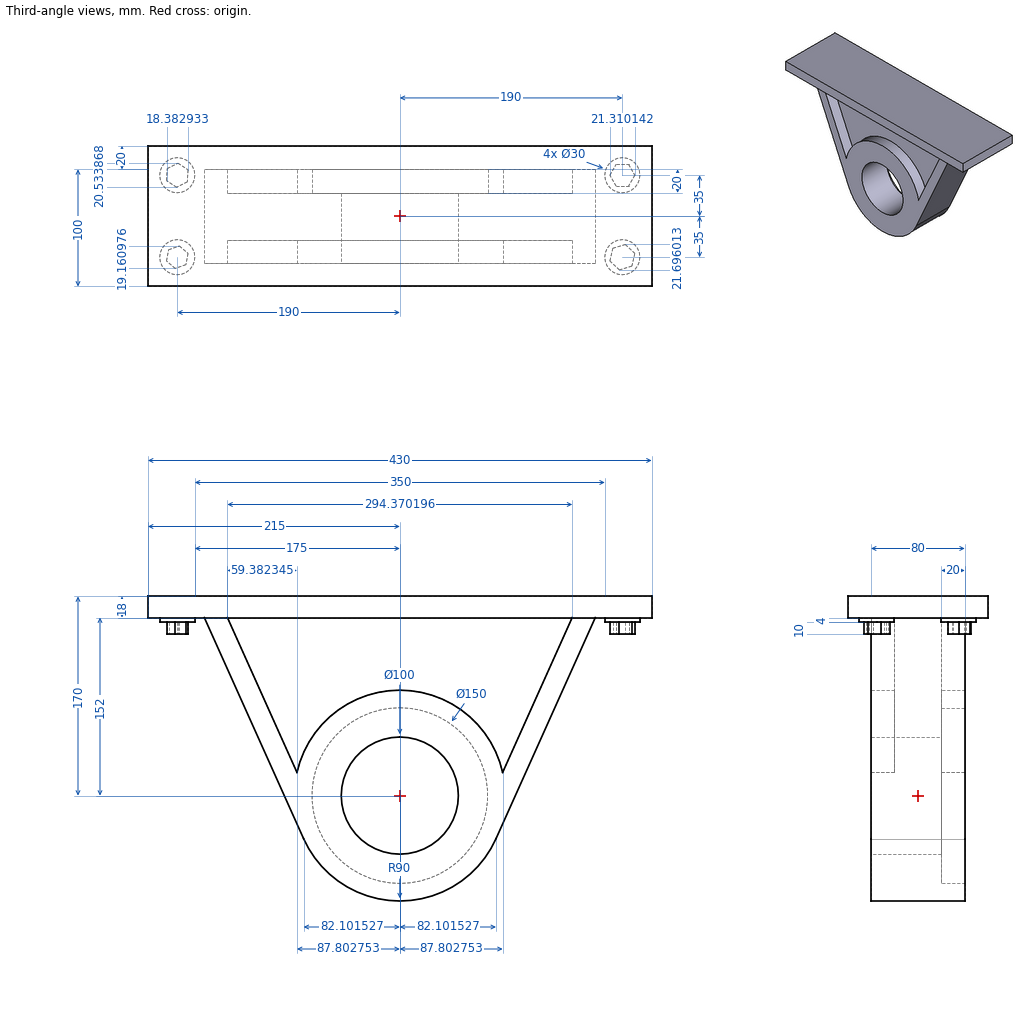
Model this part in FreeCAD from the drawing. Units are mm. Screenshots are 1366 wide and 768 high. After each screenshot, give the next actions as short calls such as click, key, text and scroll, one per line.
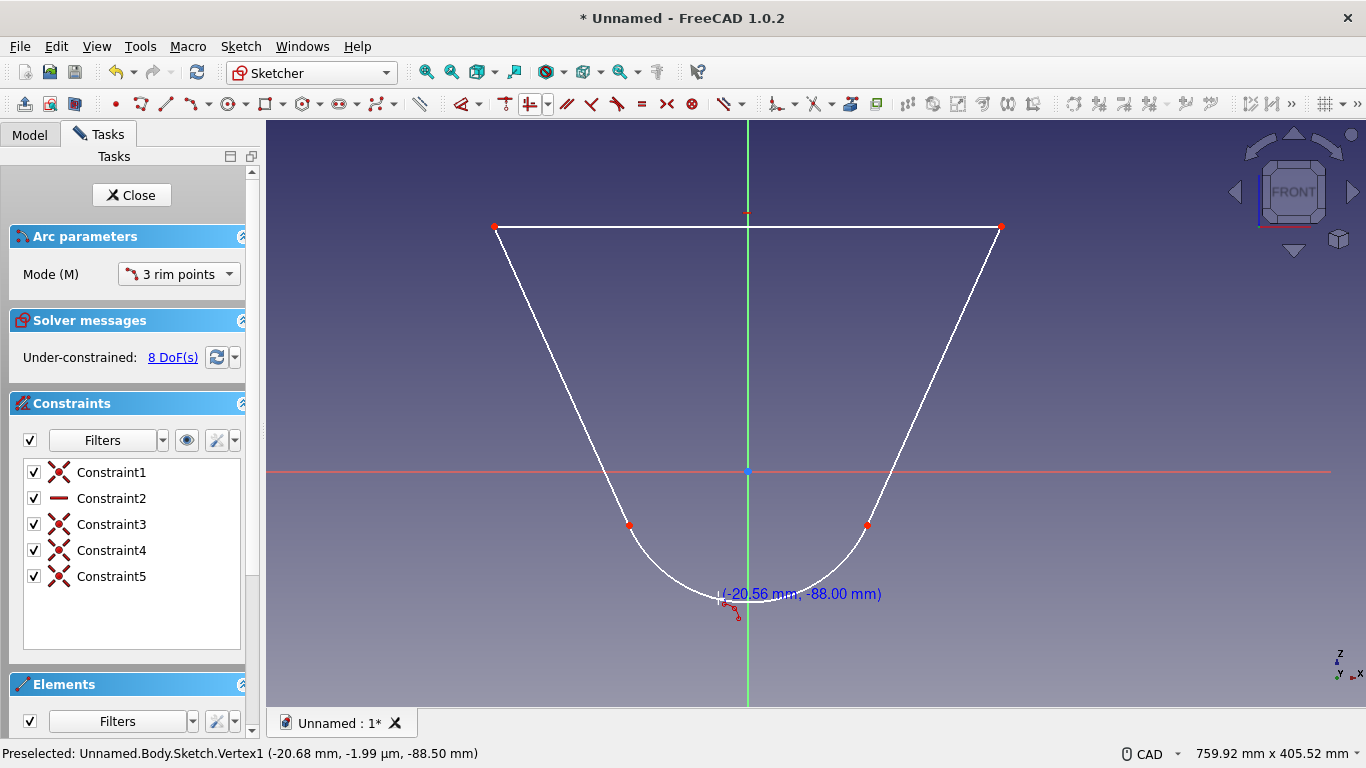
click(228, 104)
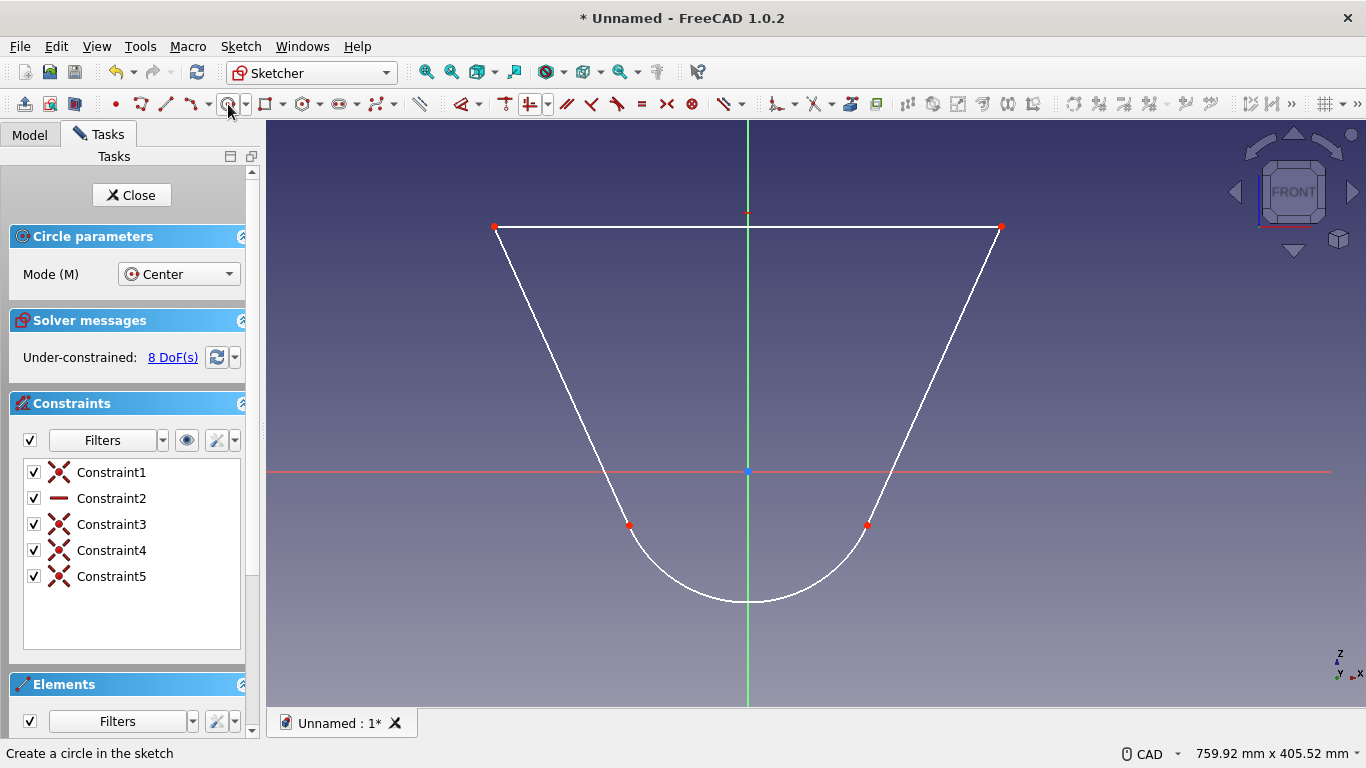
click(748, 472)
click(799, 420)
key(Escape)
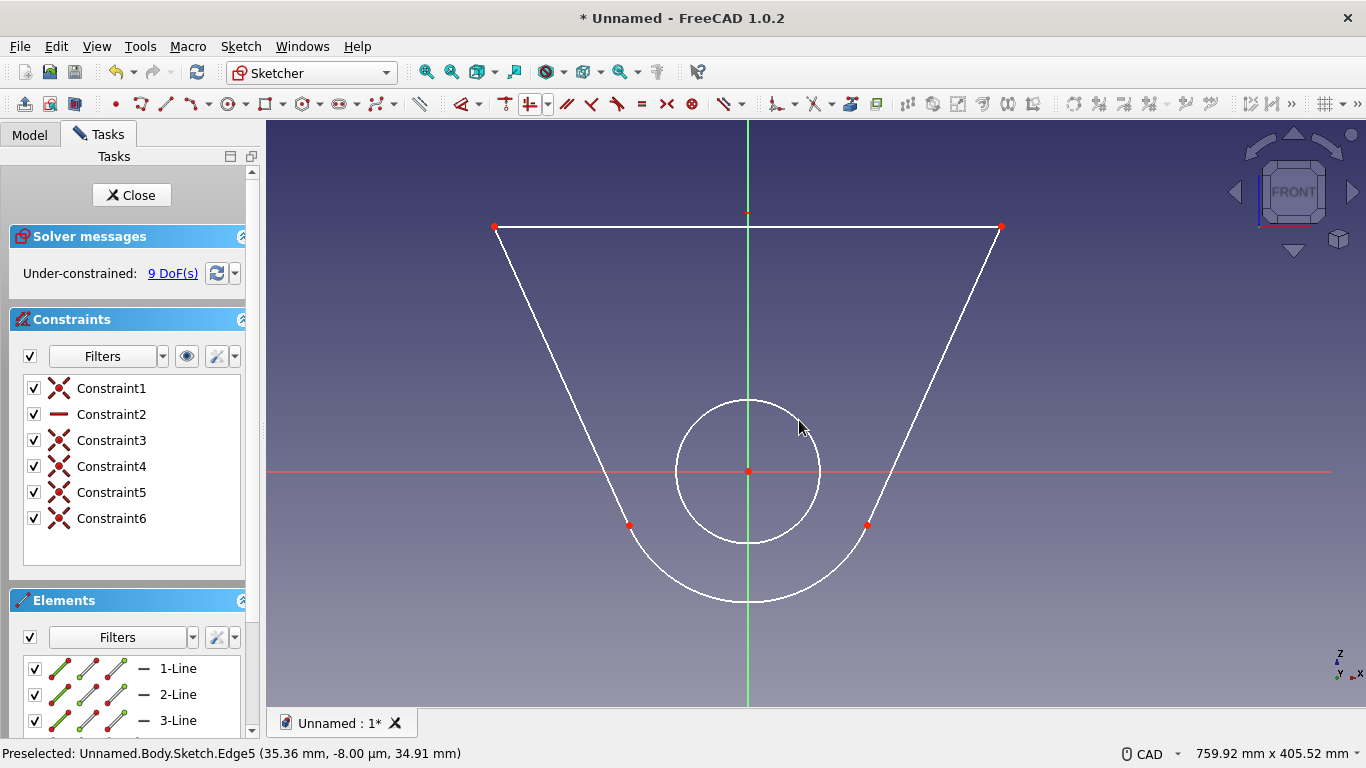
drag(738, 462, 758, 482)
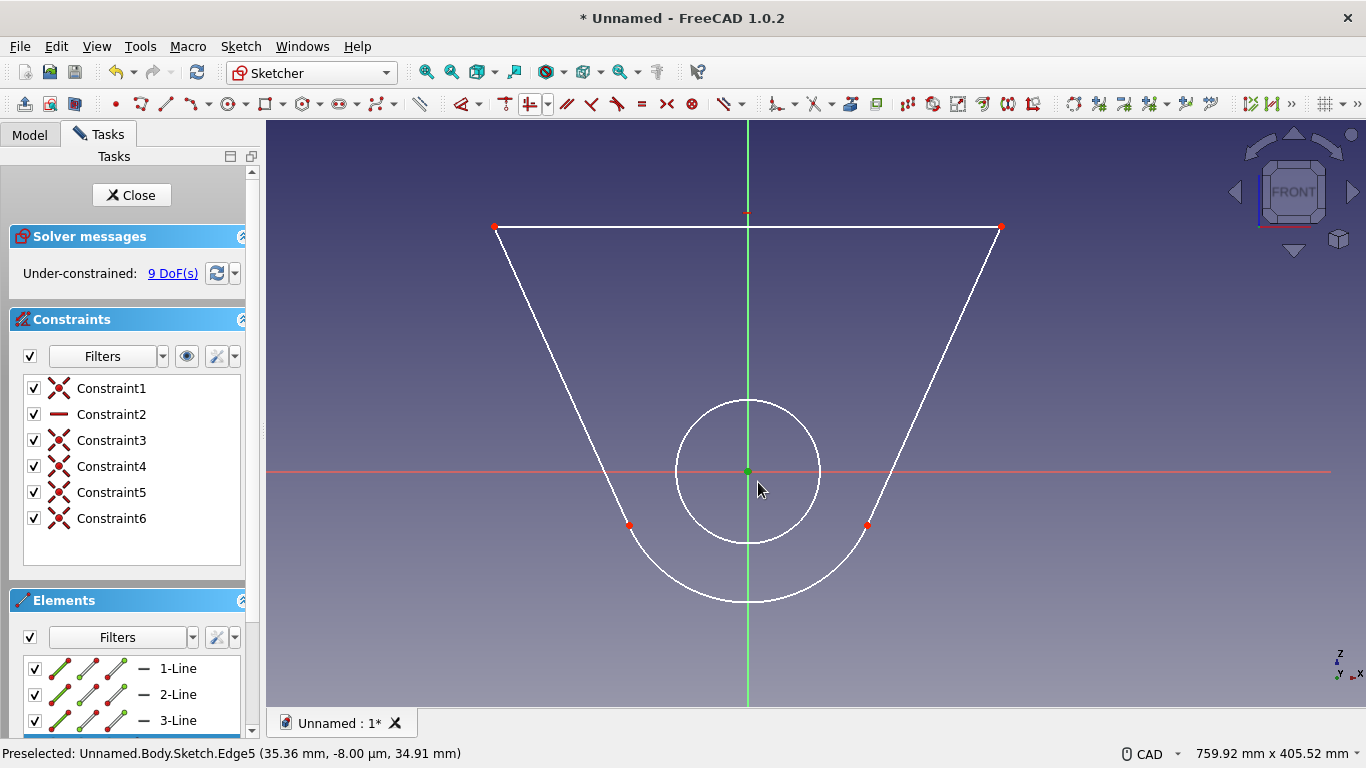
click(505, 104)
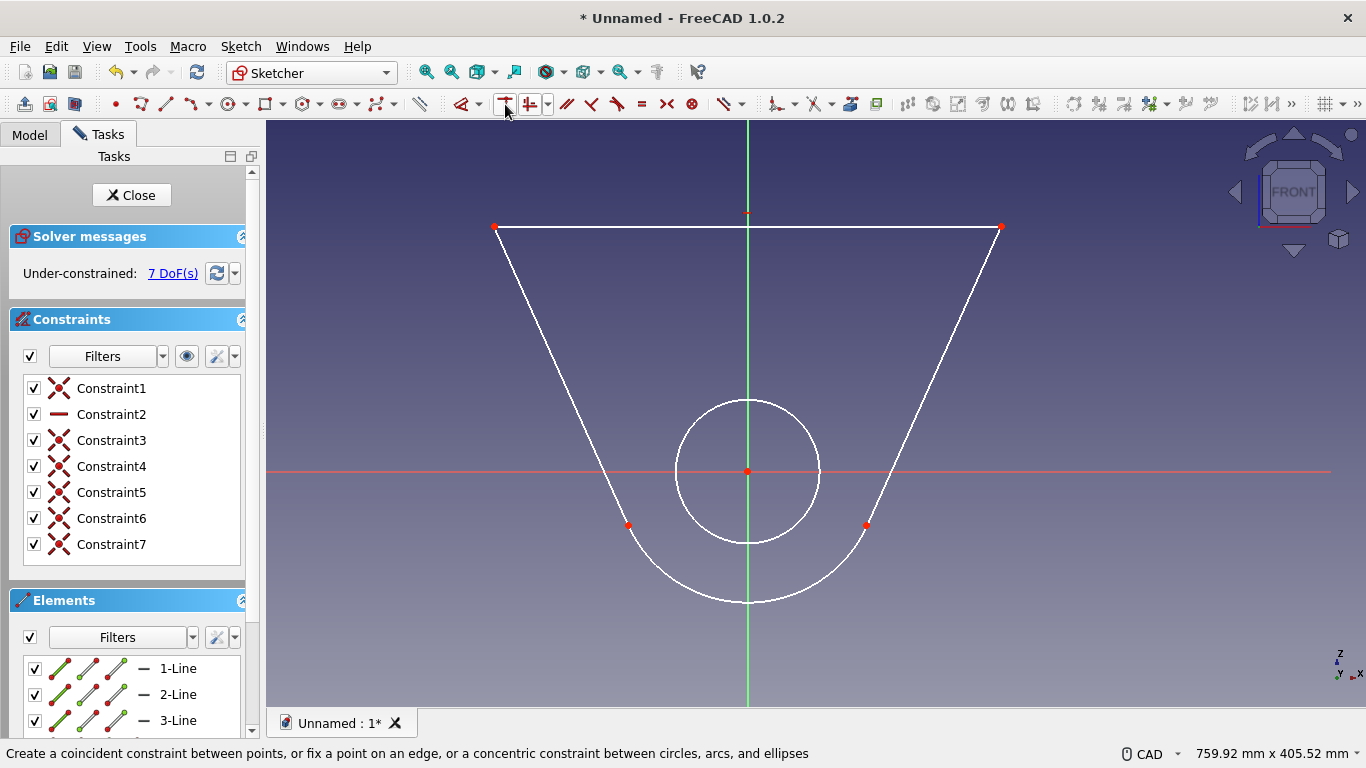
click(460, 104)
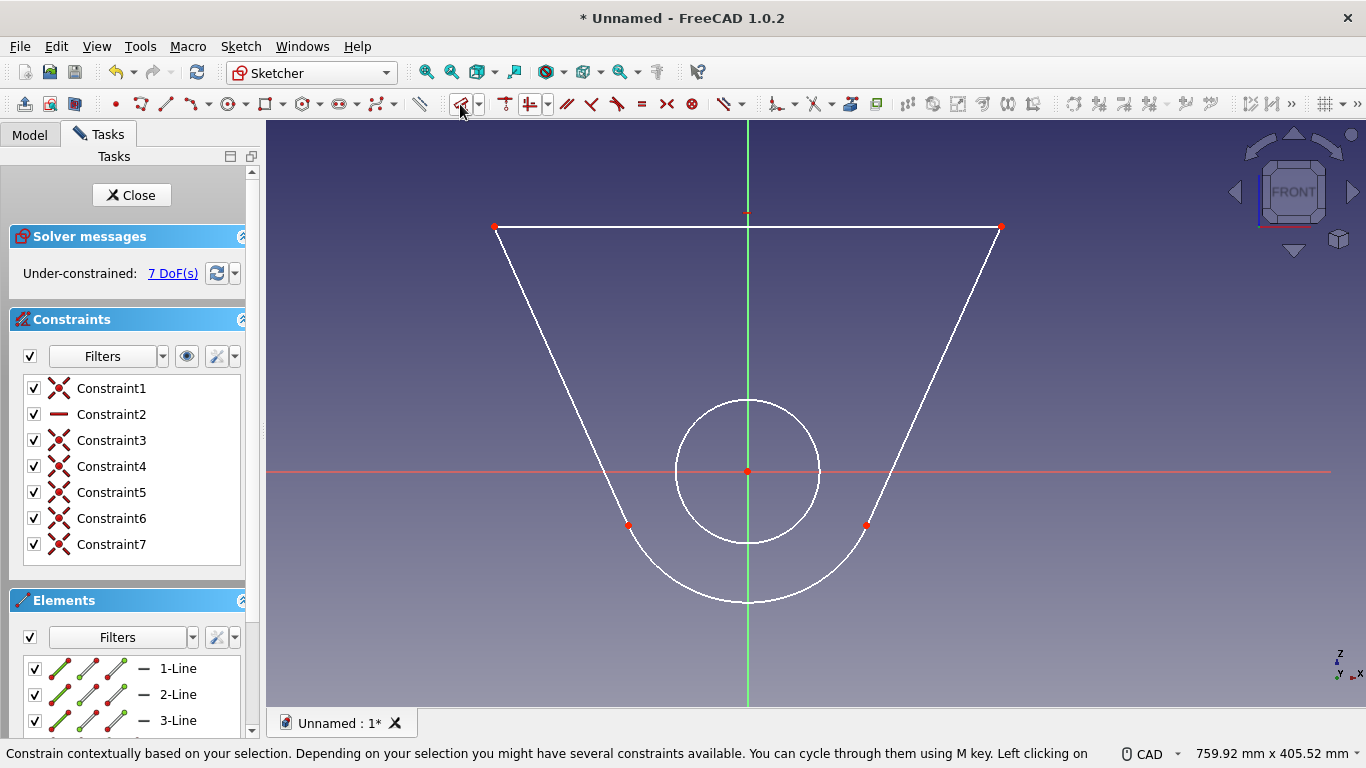
click(690, 589)
click(676, 618)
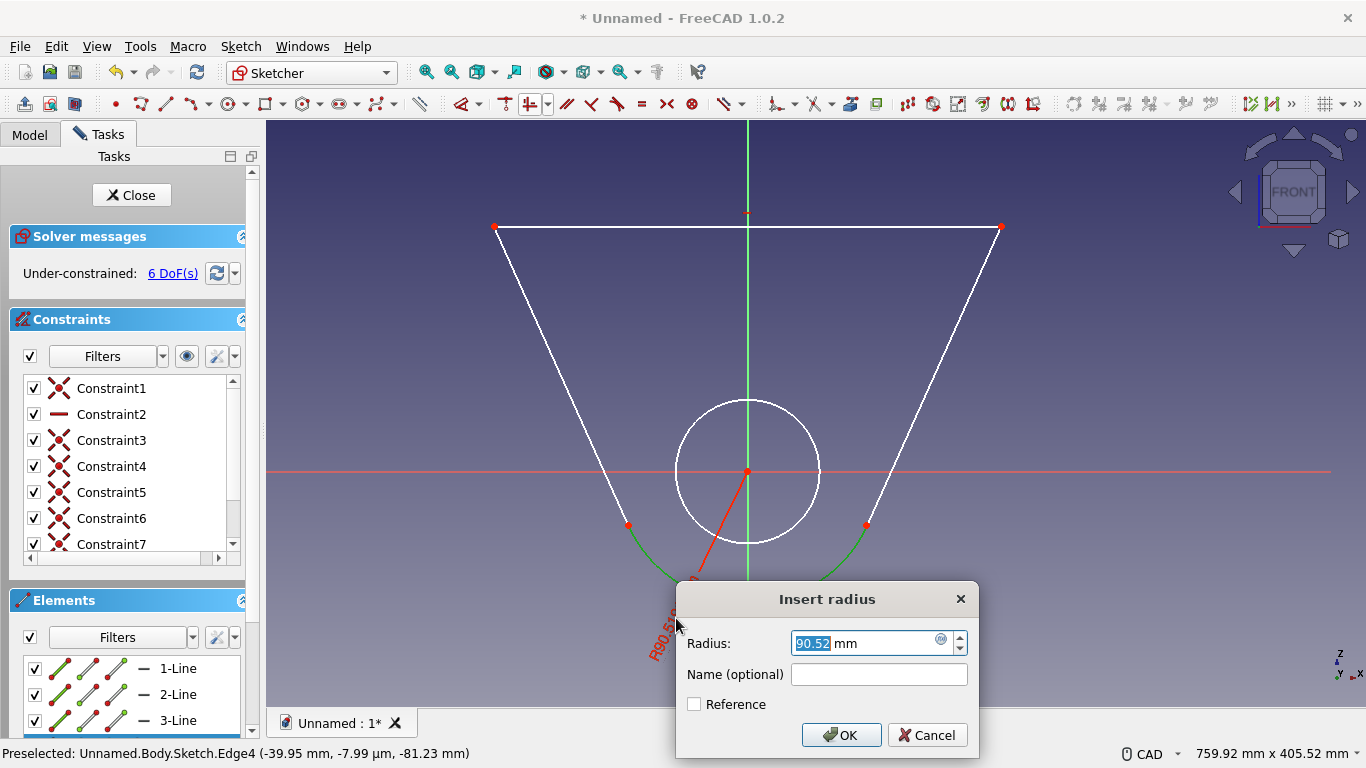
text(90)
key(Return)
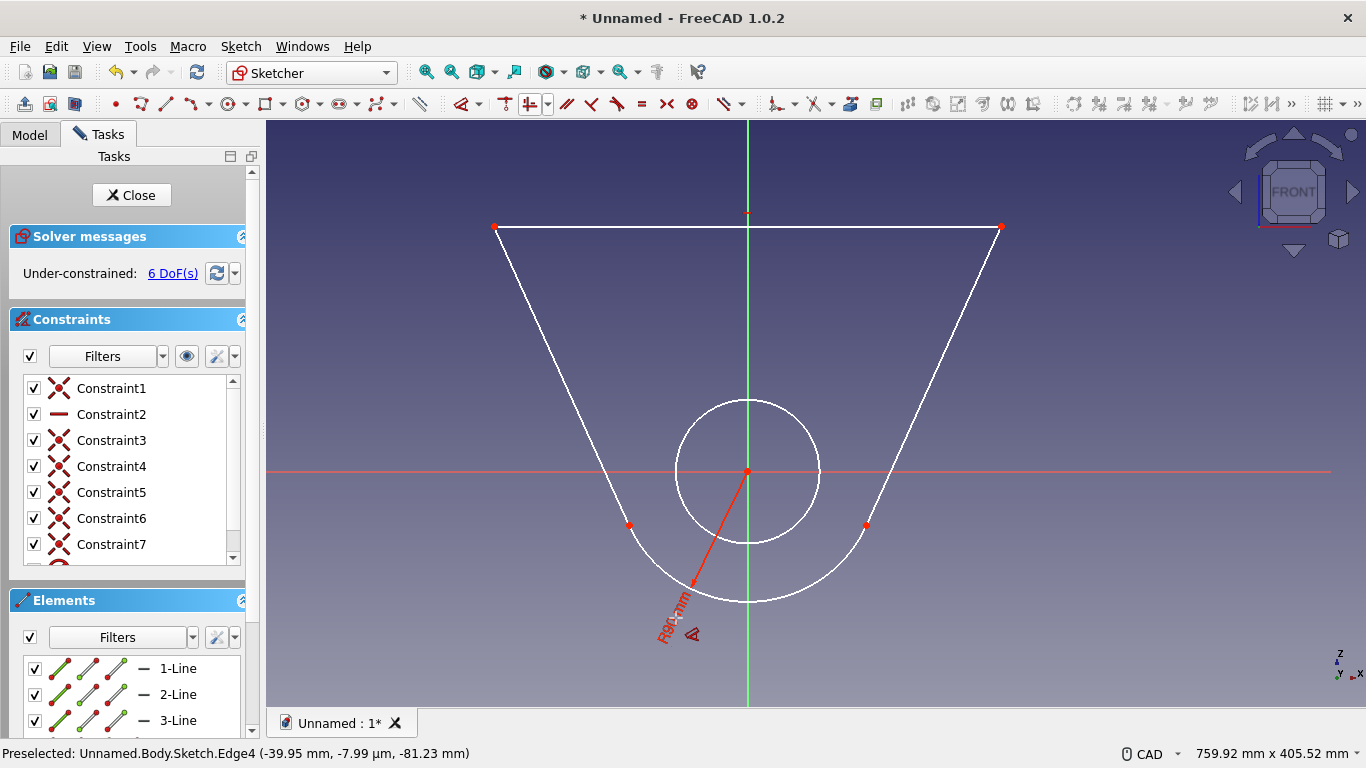
click(798, 421)
click(821, 398)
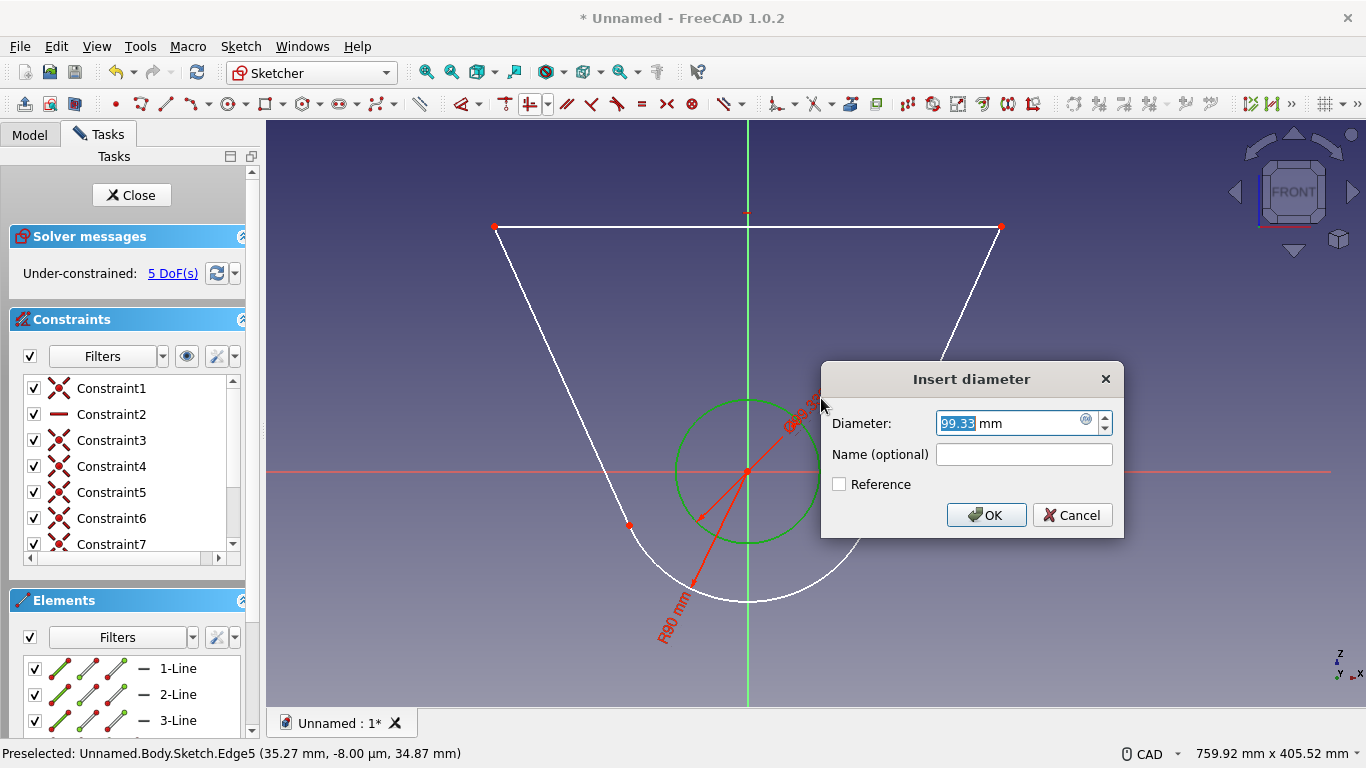
text(100)
key(Return)